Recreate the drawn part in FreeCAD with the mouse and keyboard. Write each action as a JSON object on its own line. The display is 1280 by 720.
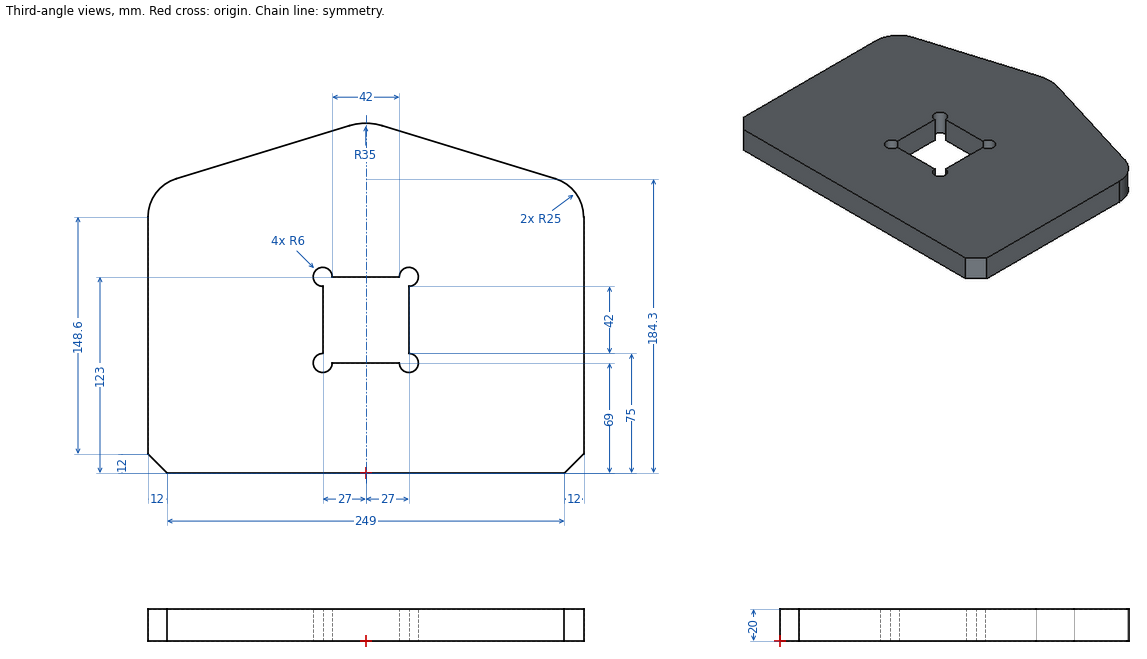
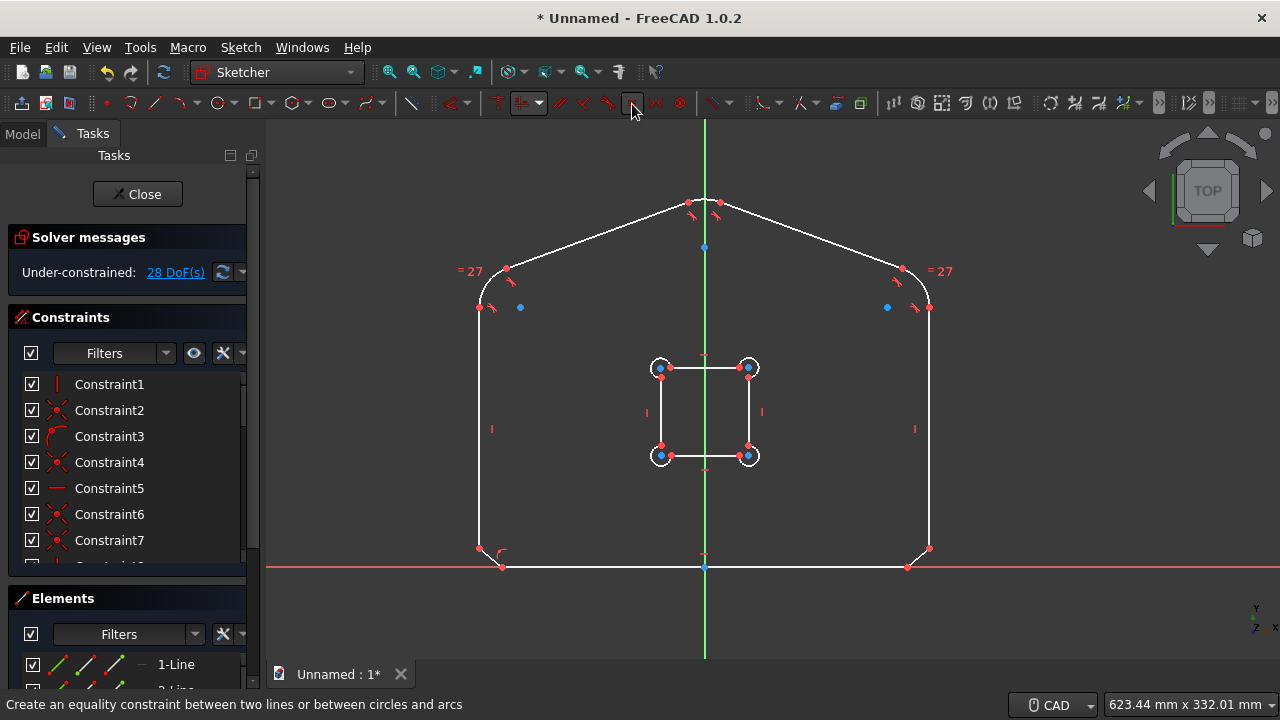
{"action": "scroll", "coordinate": [759, 369], "scroll_direction": "up", "scroll_amount": 2}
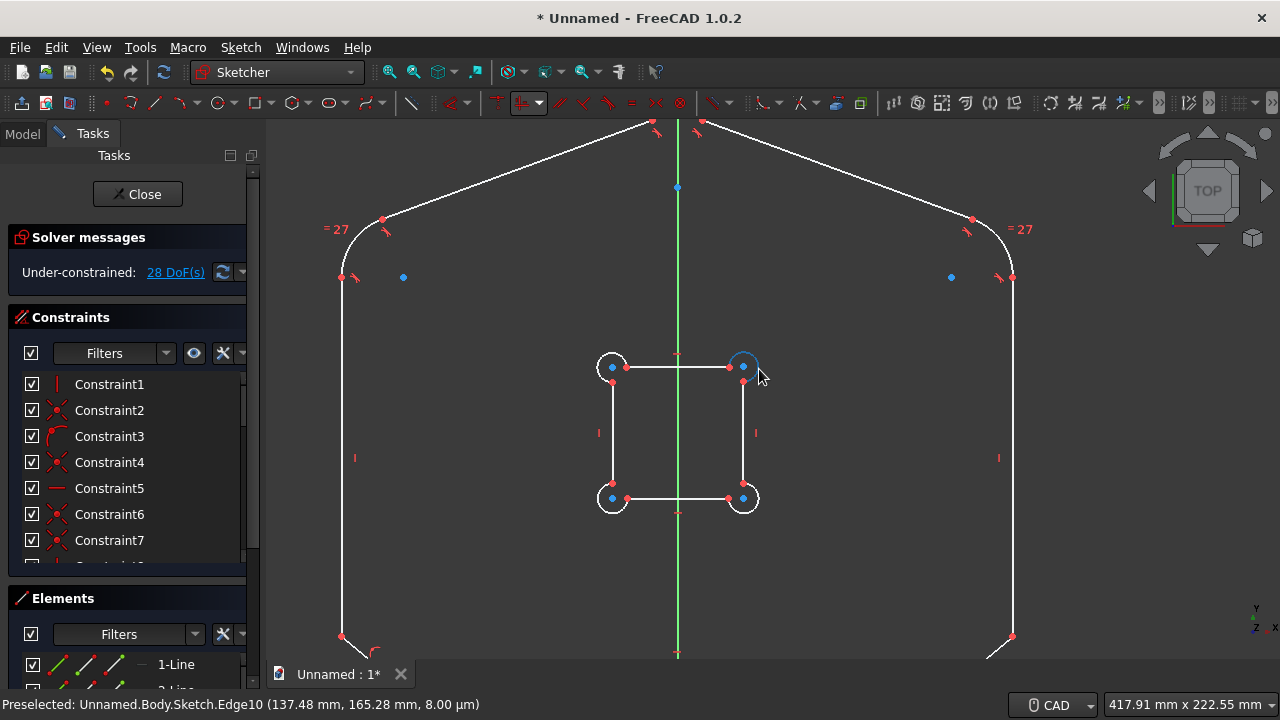
{"action": "left_click", "coordinate": [758, 369]}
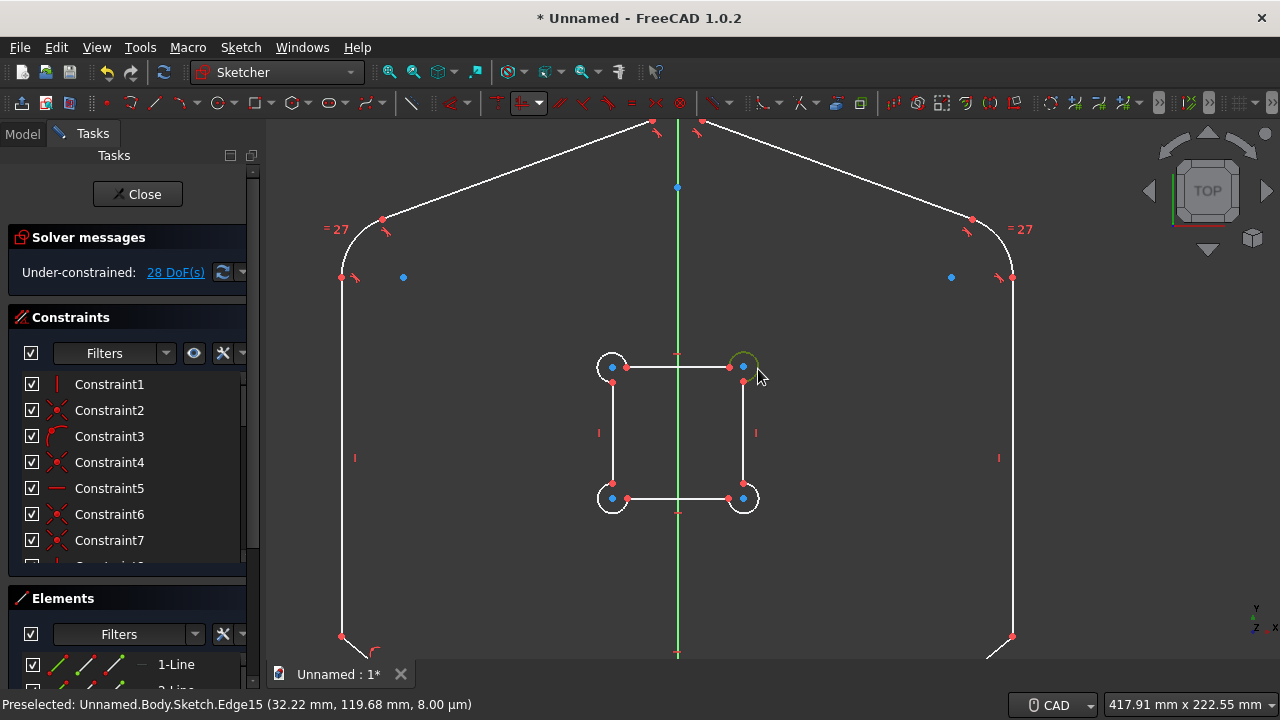
{"action": "left_click", "coordinate": [742, 513]}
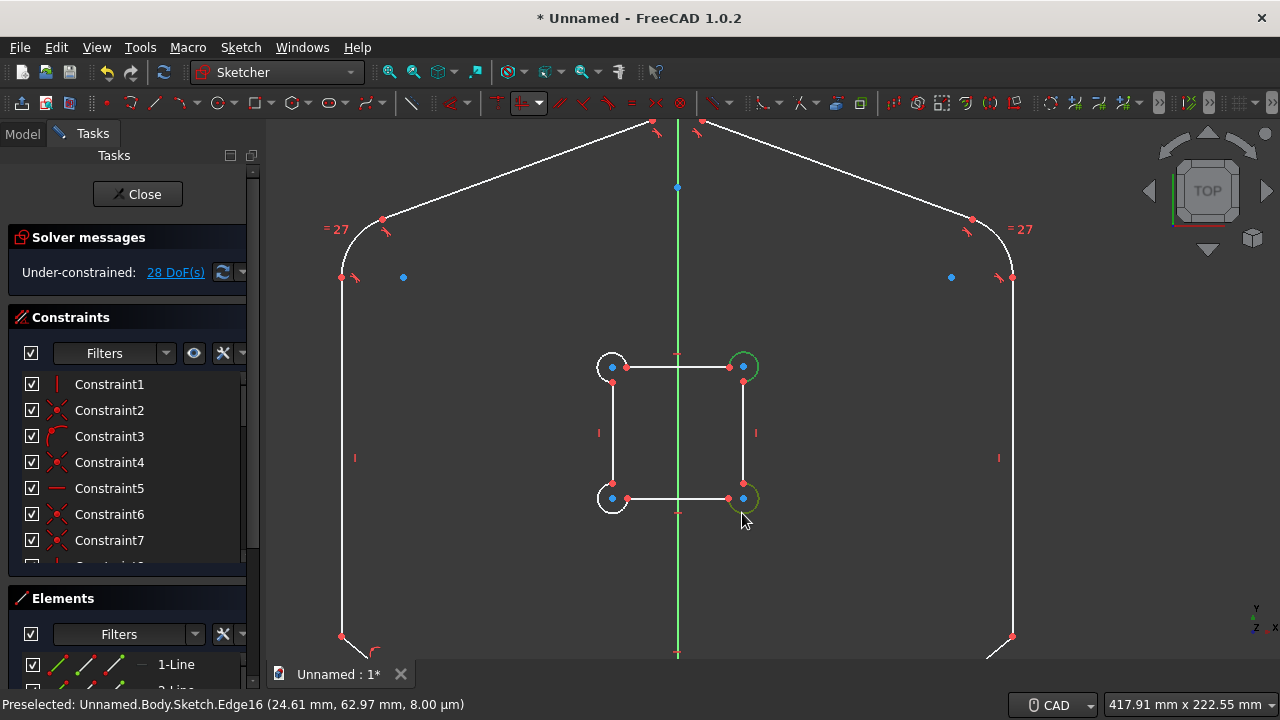
{"action": "left_click", "coordinate": [598, 496]}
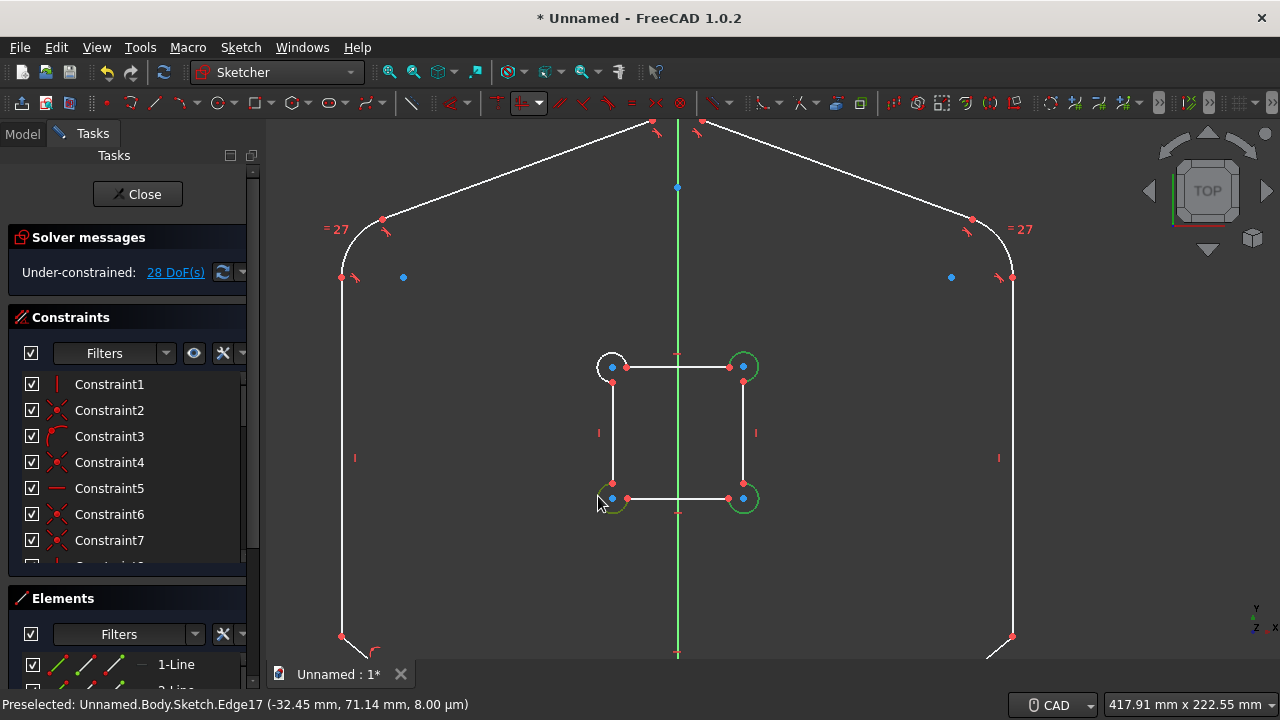
{"action": "left_click", "coordinate": [614, 353]}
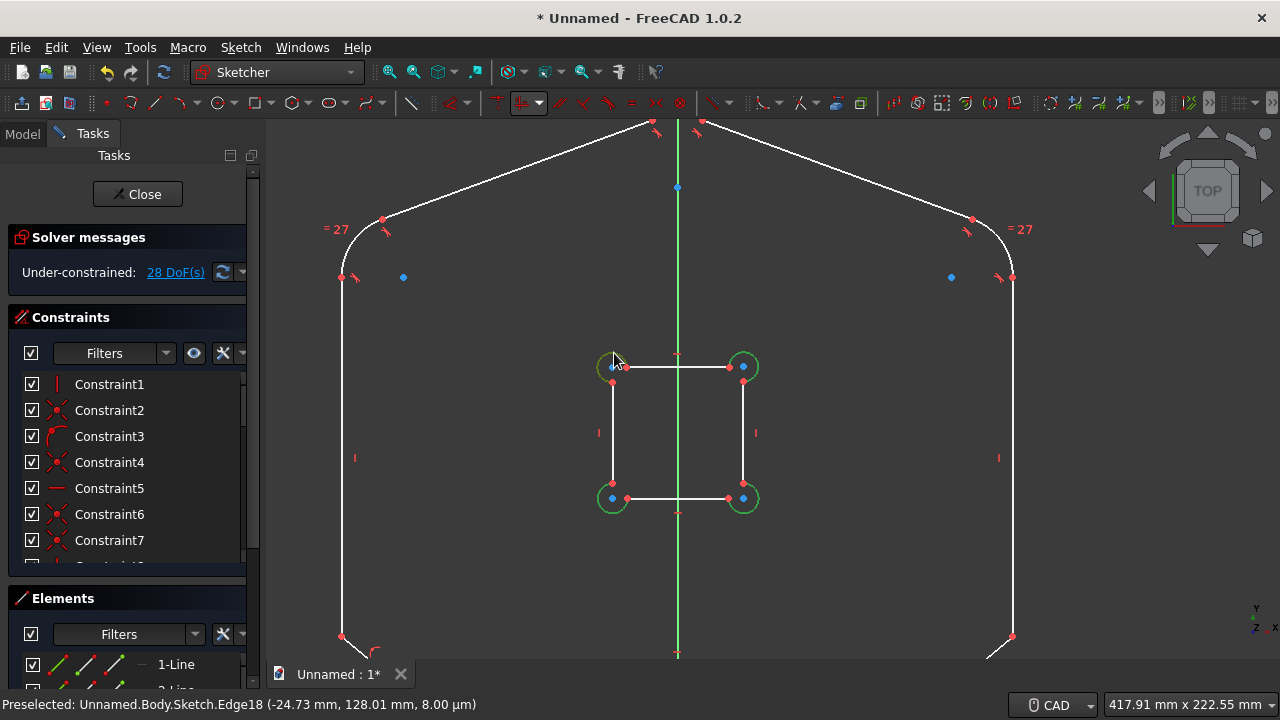
{"action": "left_click", "coordinate": [632, 104]}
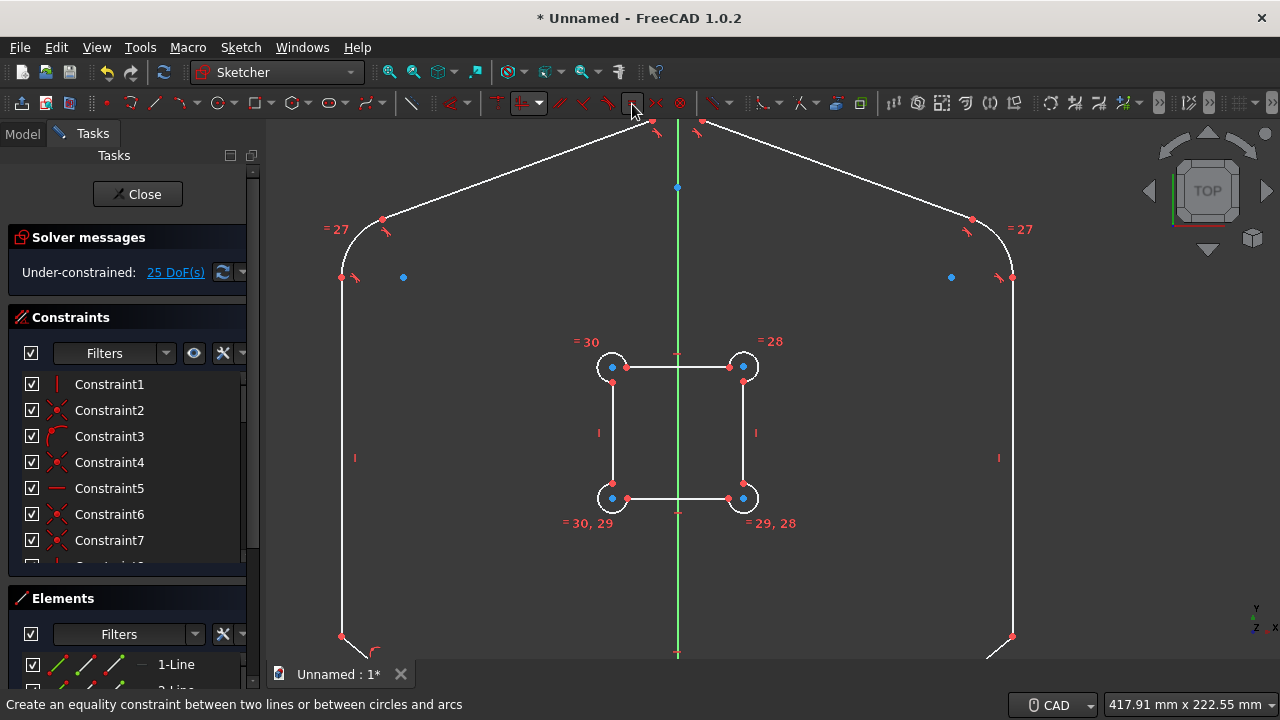
{"action": "left_click", "coordinate": [677, 187]}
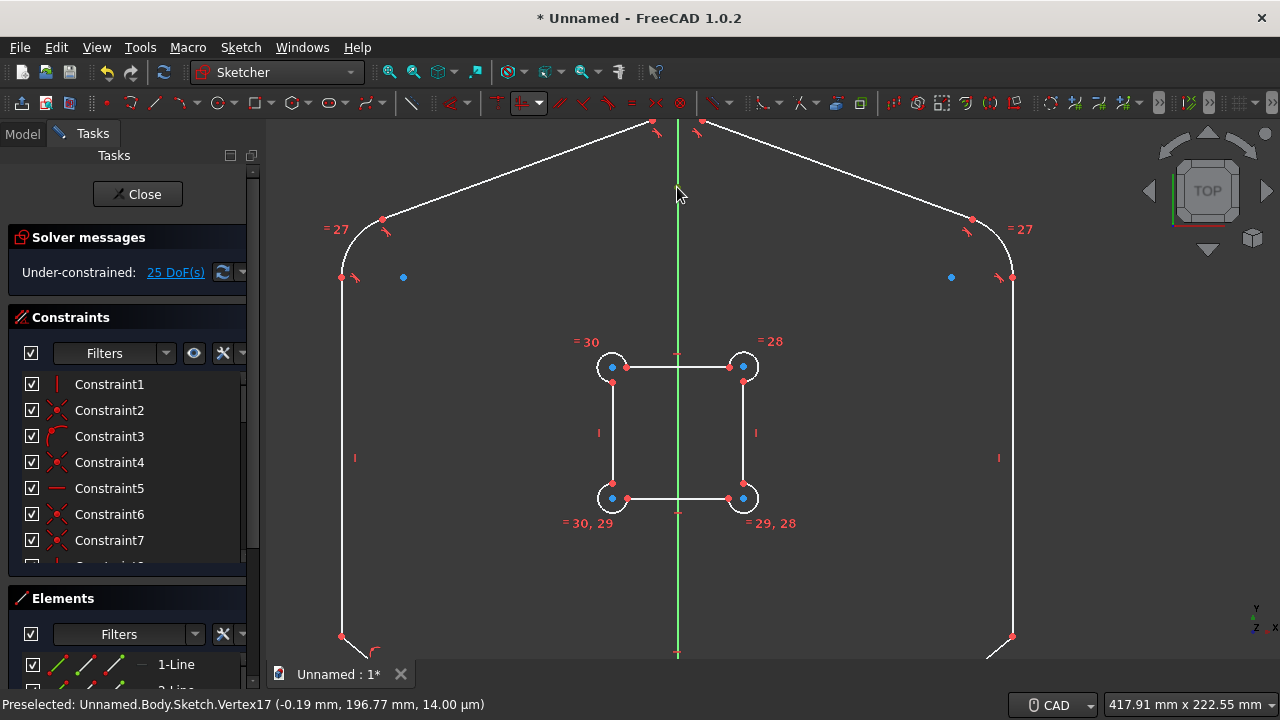
{"action": "left_click", "coordinate": [678, 596]}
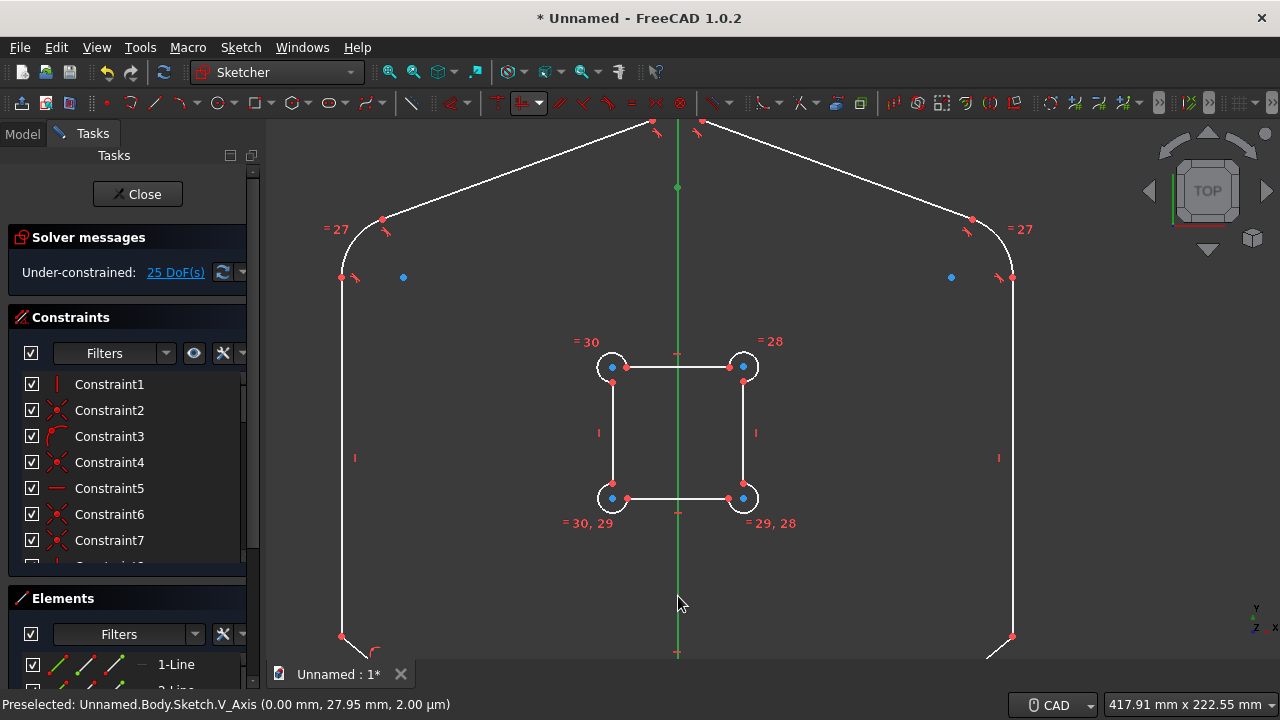
{"action": "left_click", "coordinate": [498, 104]}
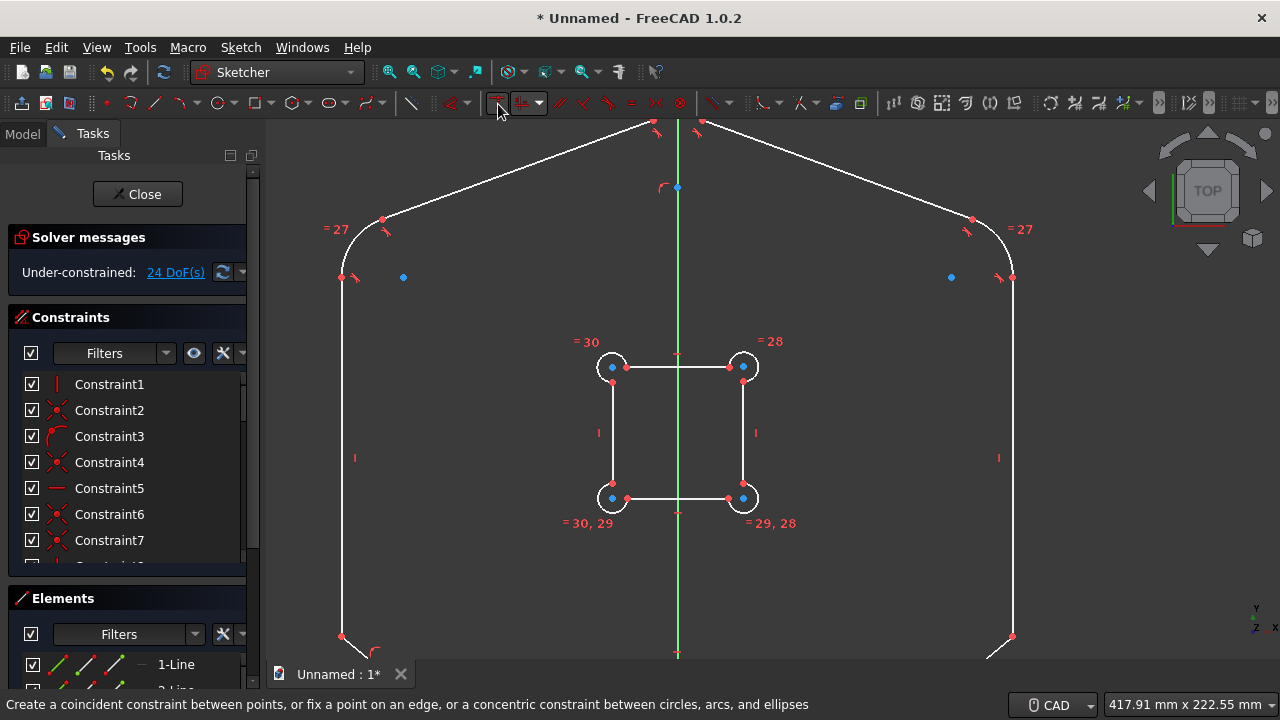
{"action": "left_click", "coordinate": [404, 277]}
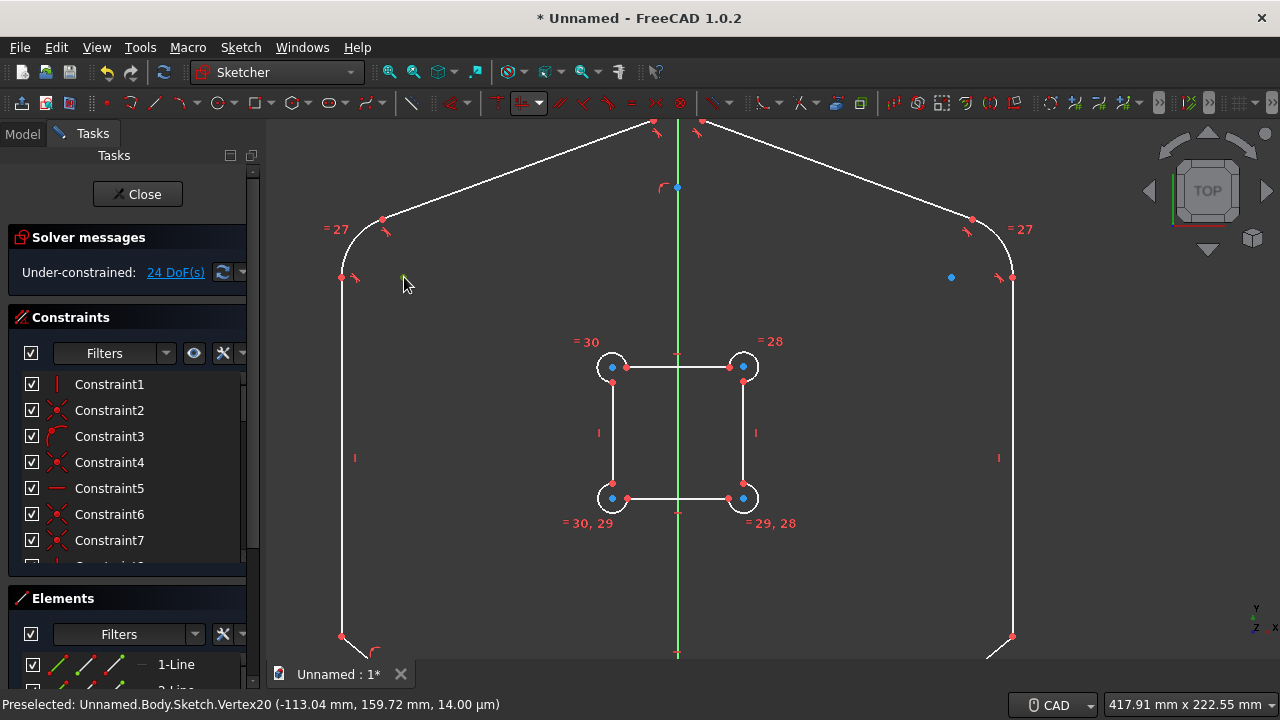
{"action": "left_click", "coordinate": [951, 277]}